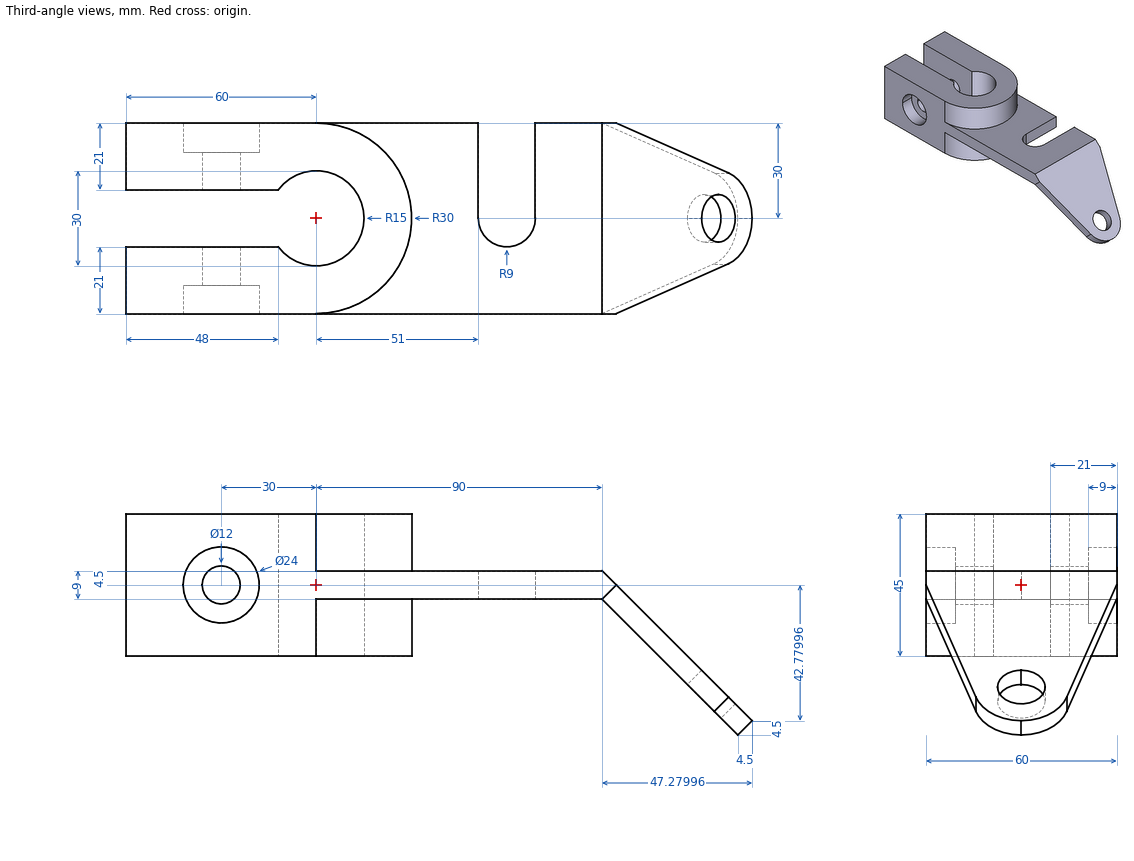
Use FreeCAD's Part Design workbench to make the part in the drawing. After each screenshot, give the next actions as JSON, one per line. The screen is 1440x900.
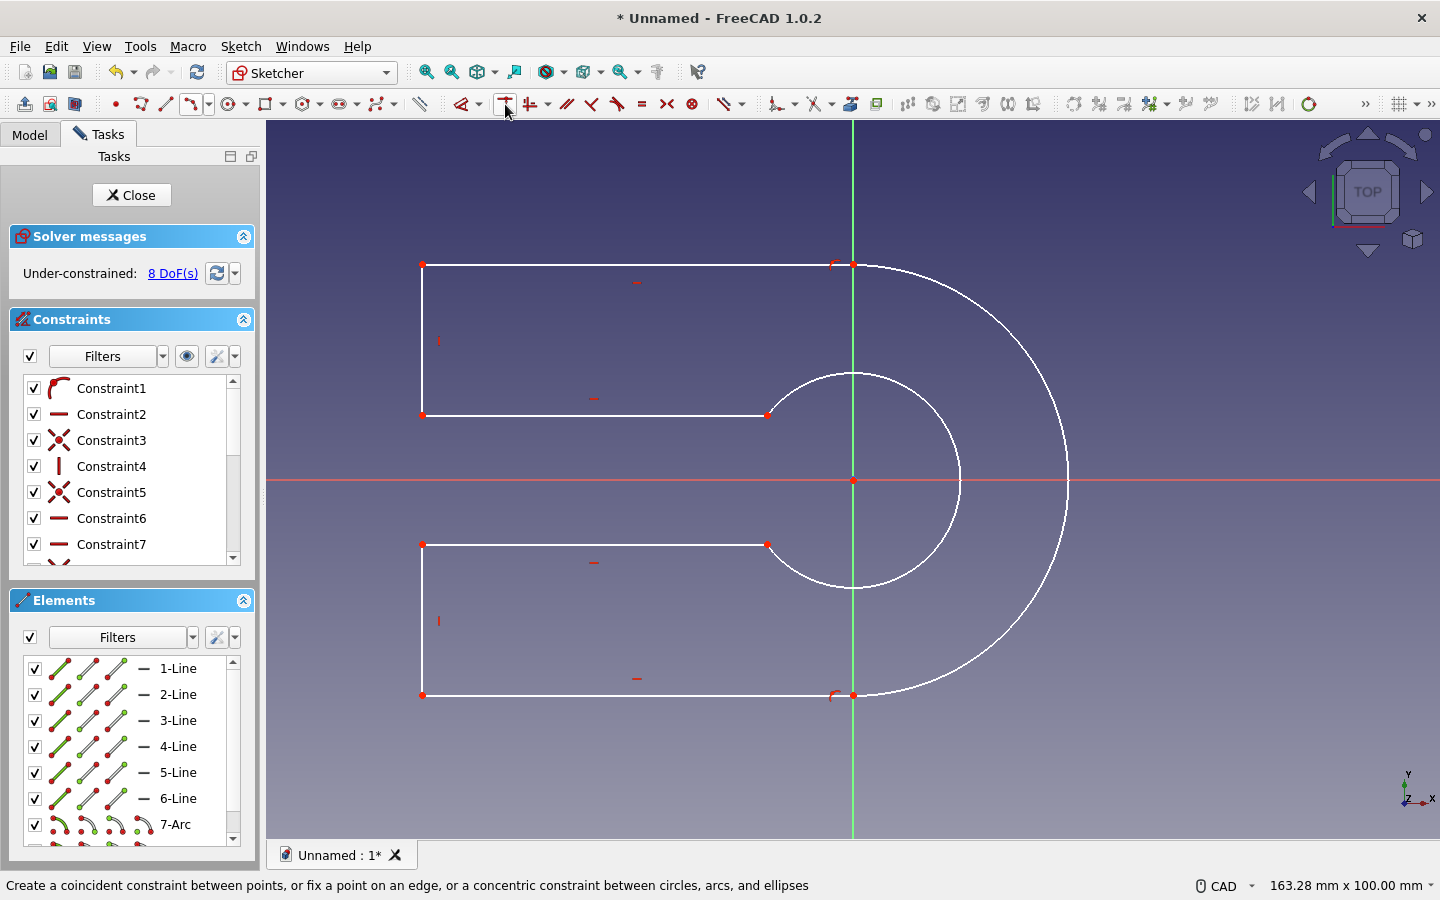
{"action": "left_click_drag", "start_coordinate": [843, 470], "coordinate": [863, 490]}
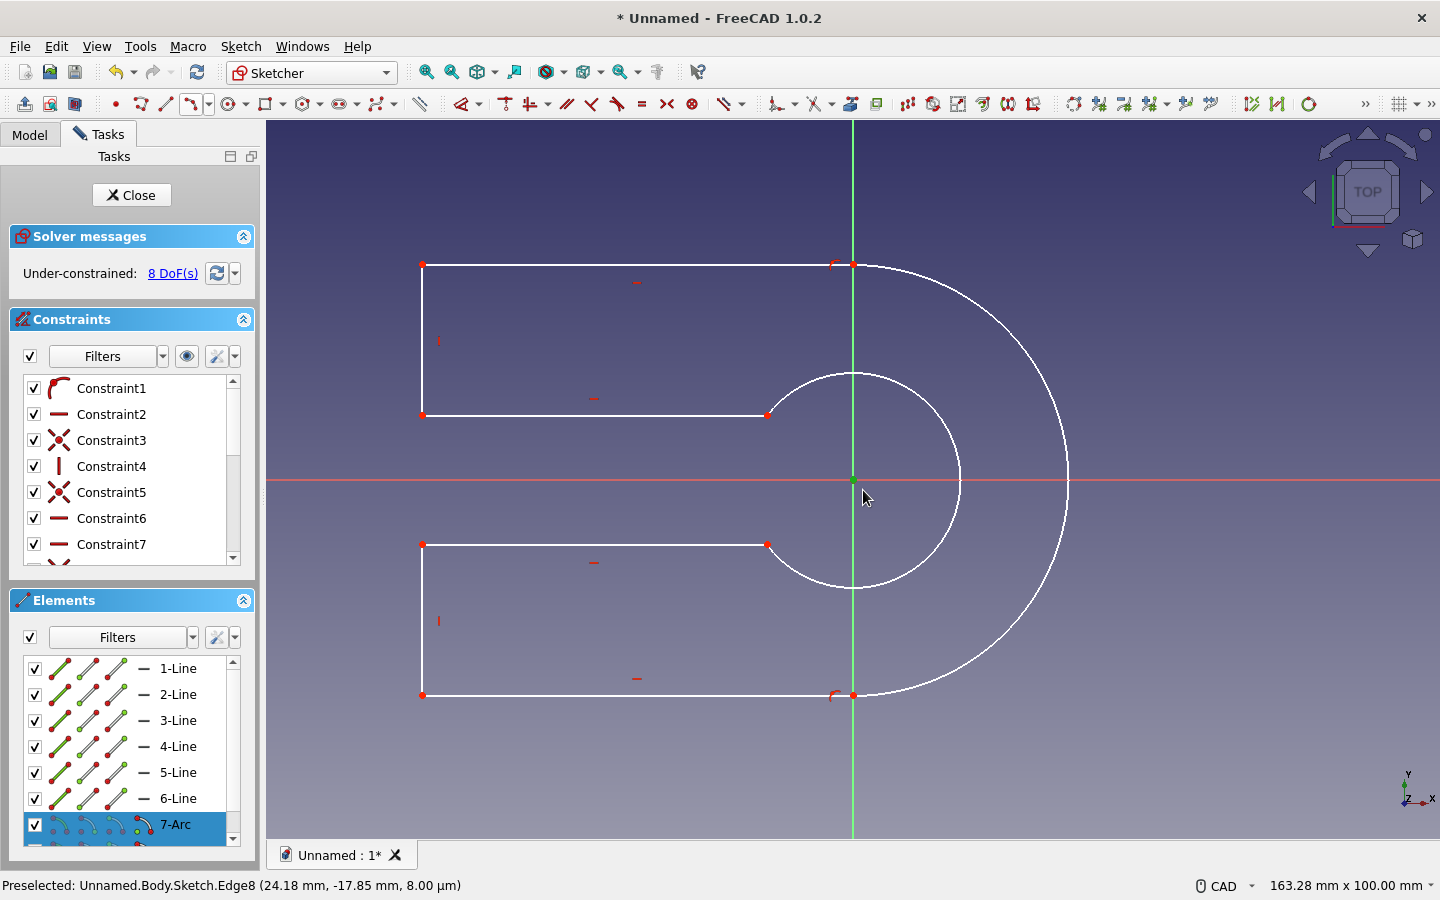
{"action": "left_click", "coordinate": [505, 104]}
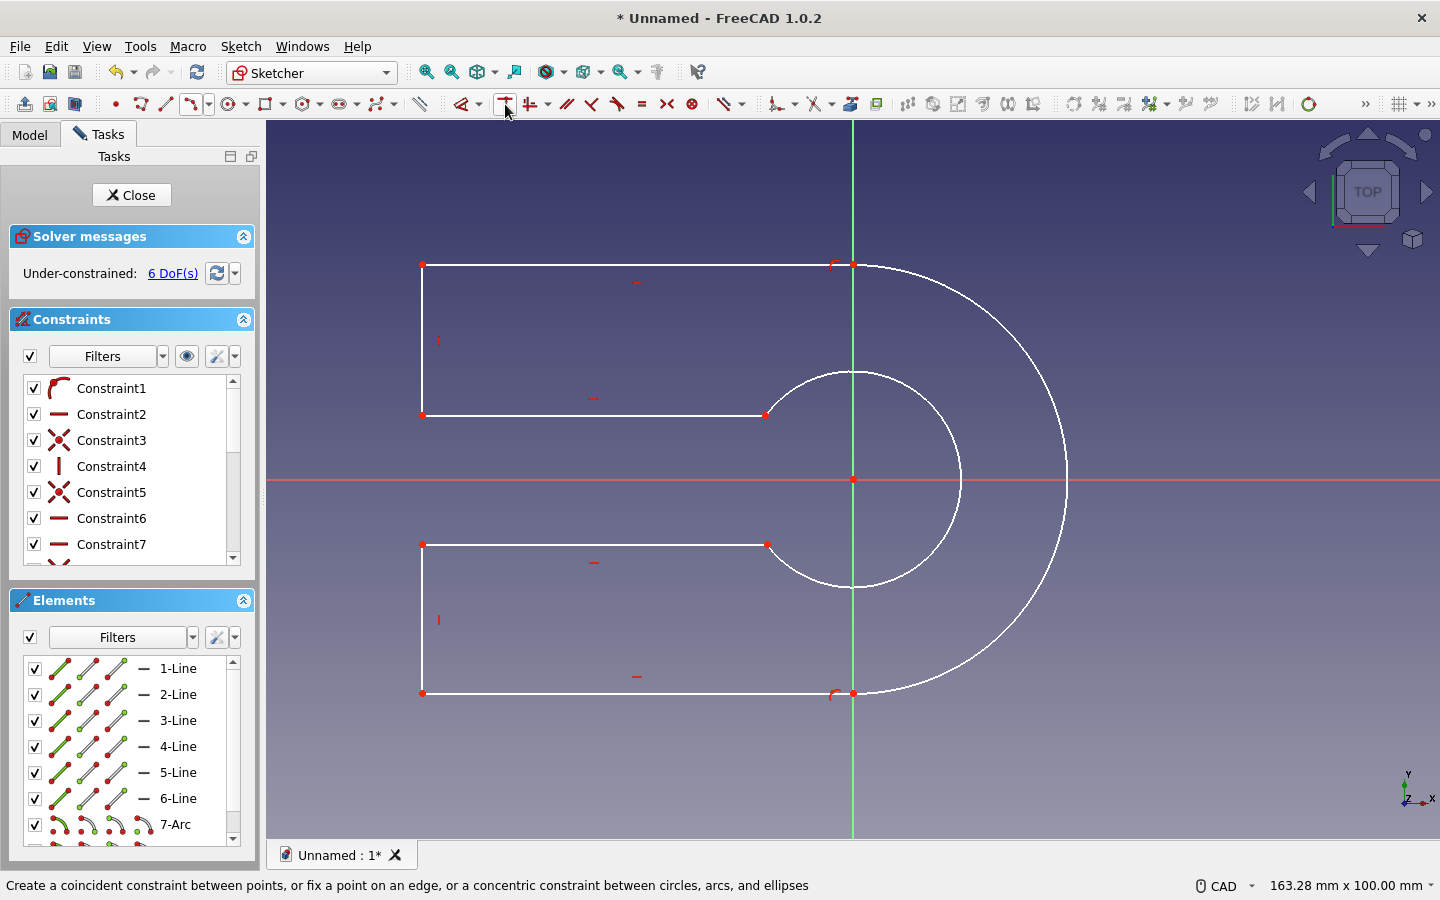
{"action": "left_click", "coordinate": [912, 570]}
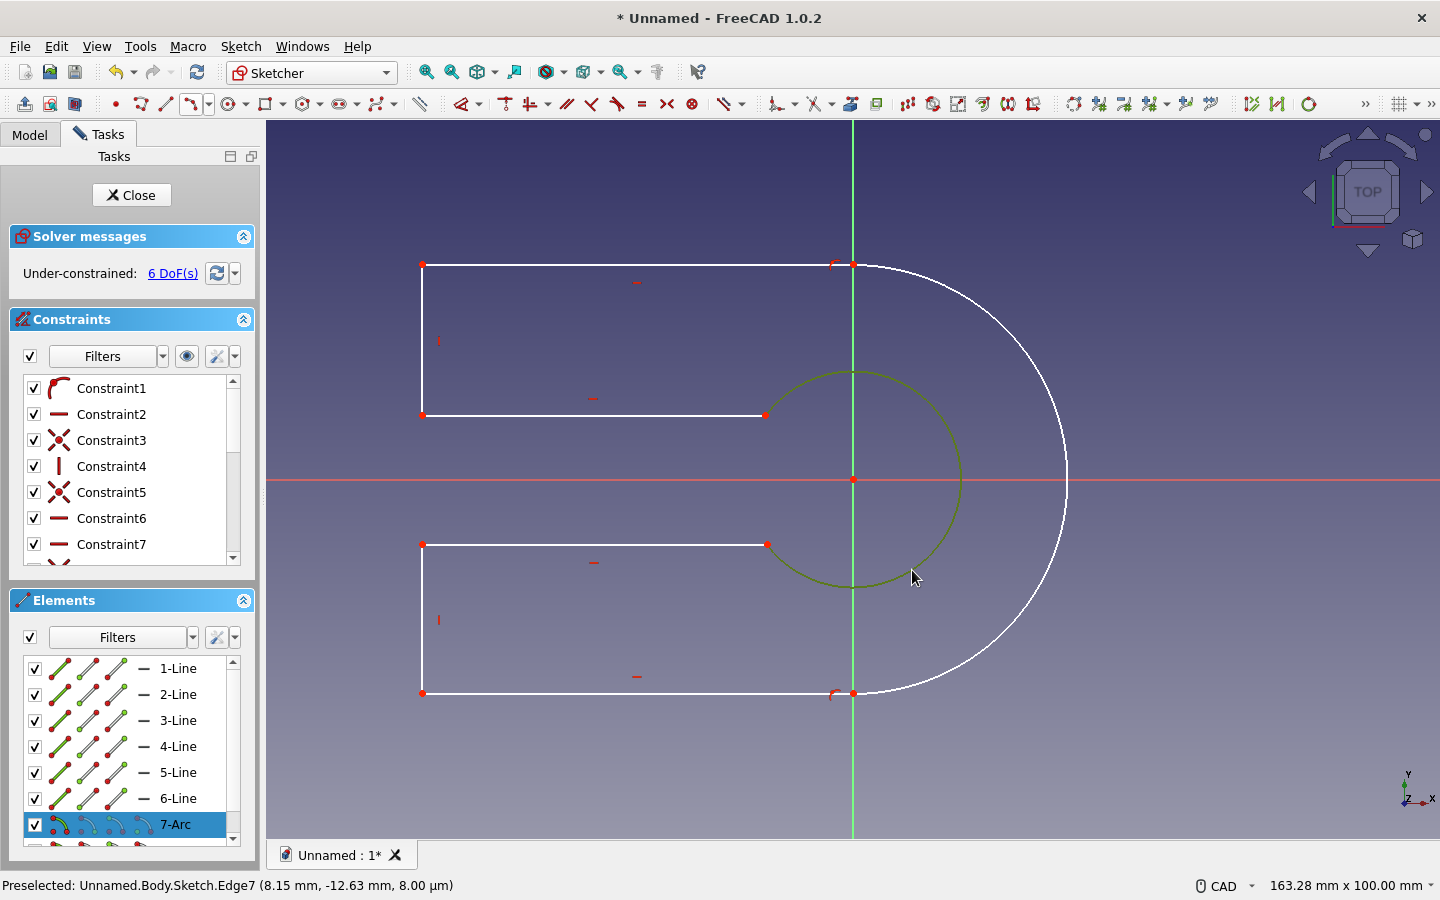
{"action": "left_click", "coordinate": [478, 104]}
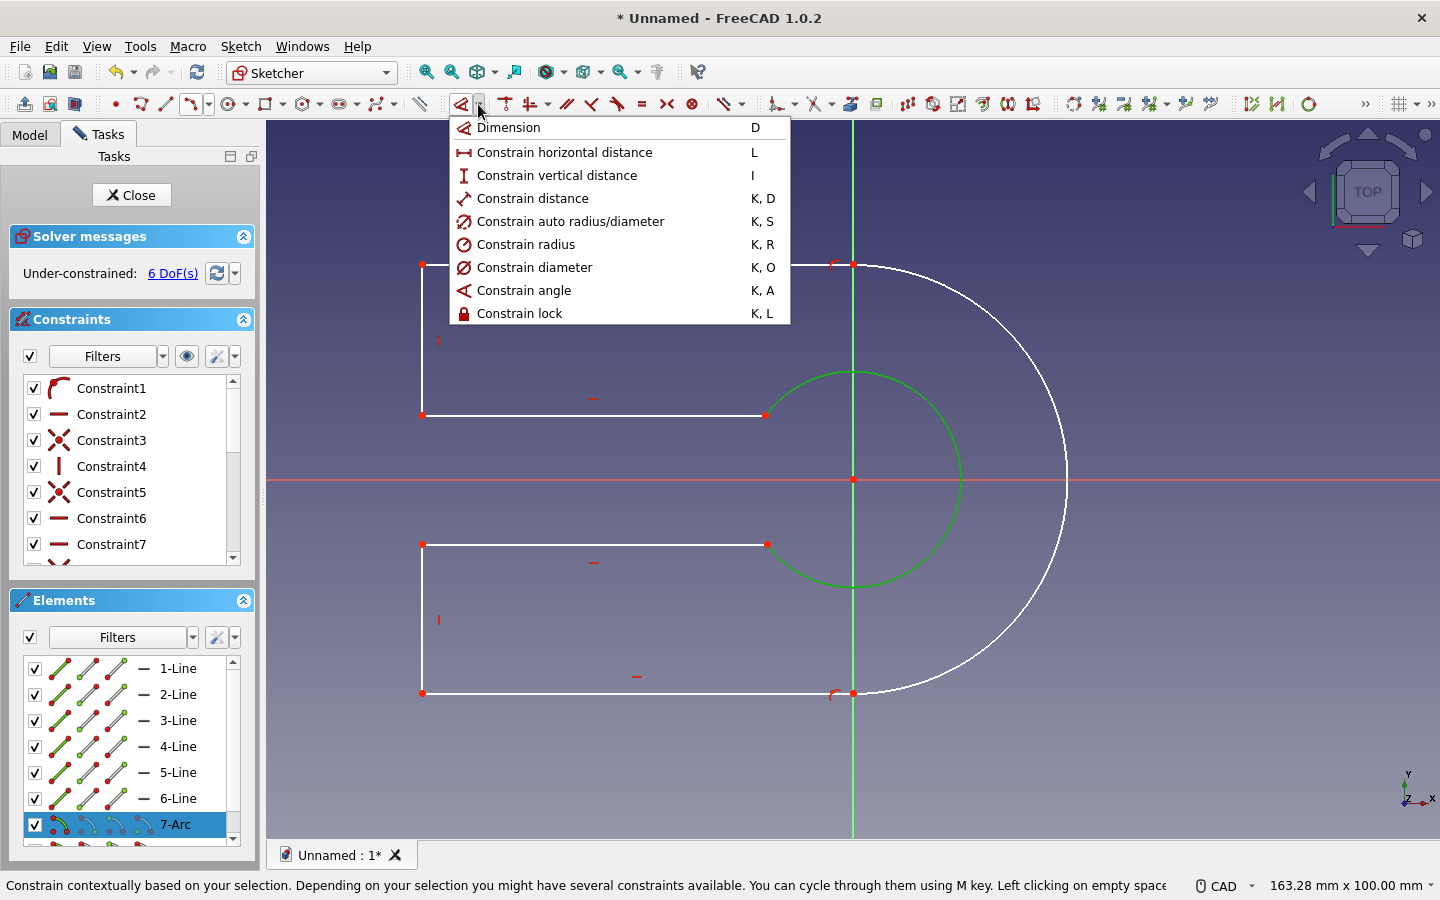
{"action": "left_click", "coordinate": [620, 244]}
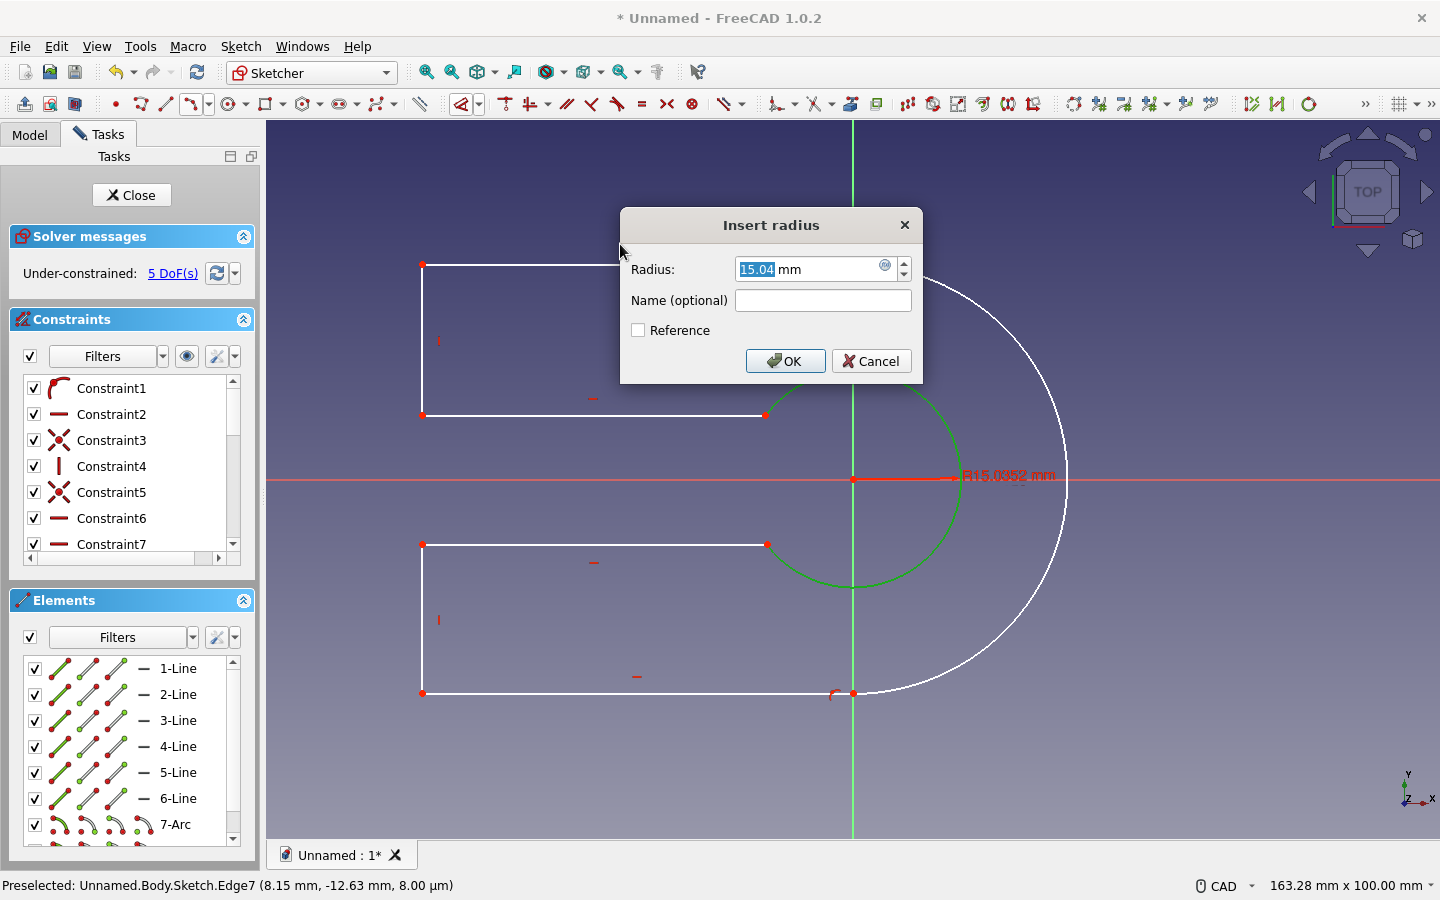
{"action": "type", "text": "15"}
{"action": "key", "text": "Return"}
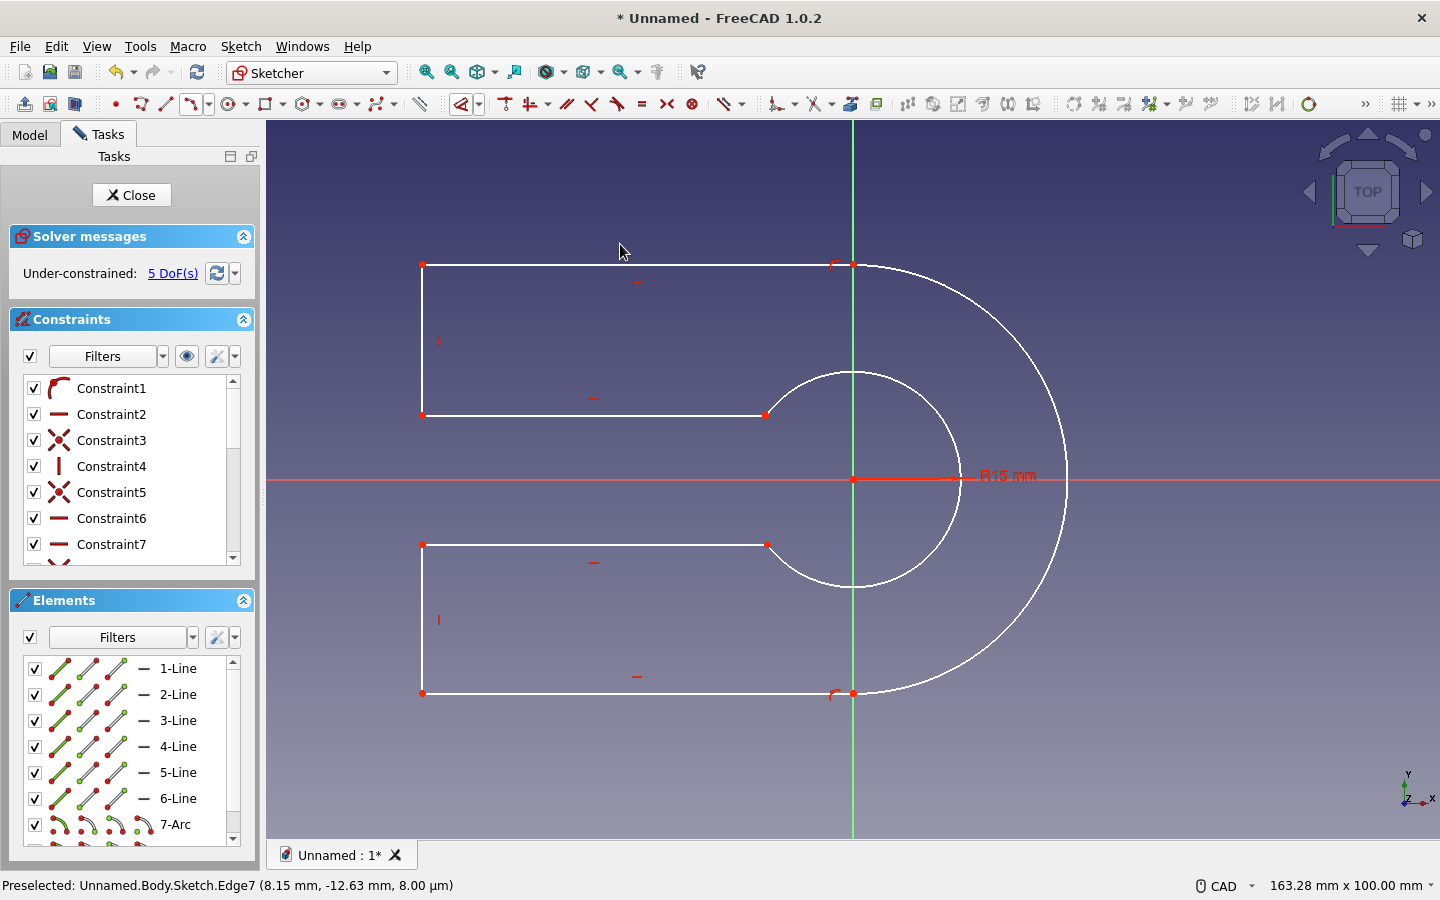
{"action": "left_click", "coordinate": [1027, 606]}